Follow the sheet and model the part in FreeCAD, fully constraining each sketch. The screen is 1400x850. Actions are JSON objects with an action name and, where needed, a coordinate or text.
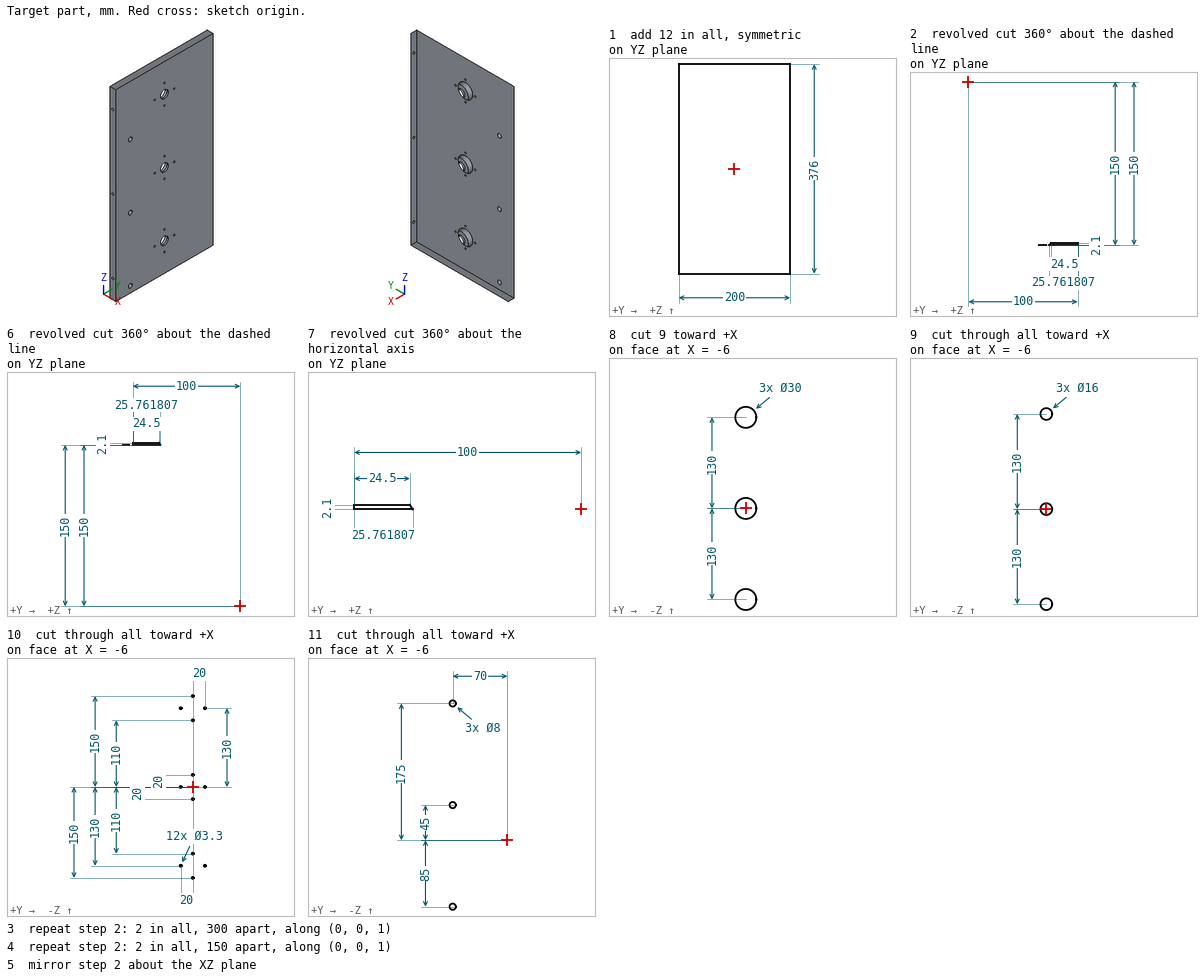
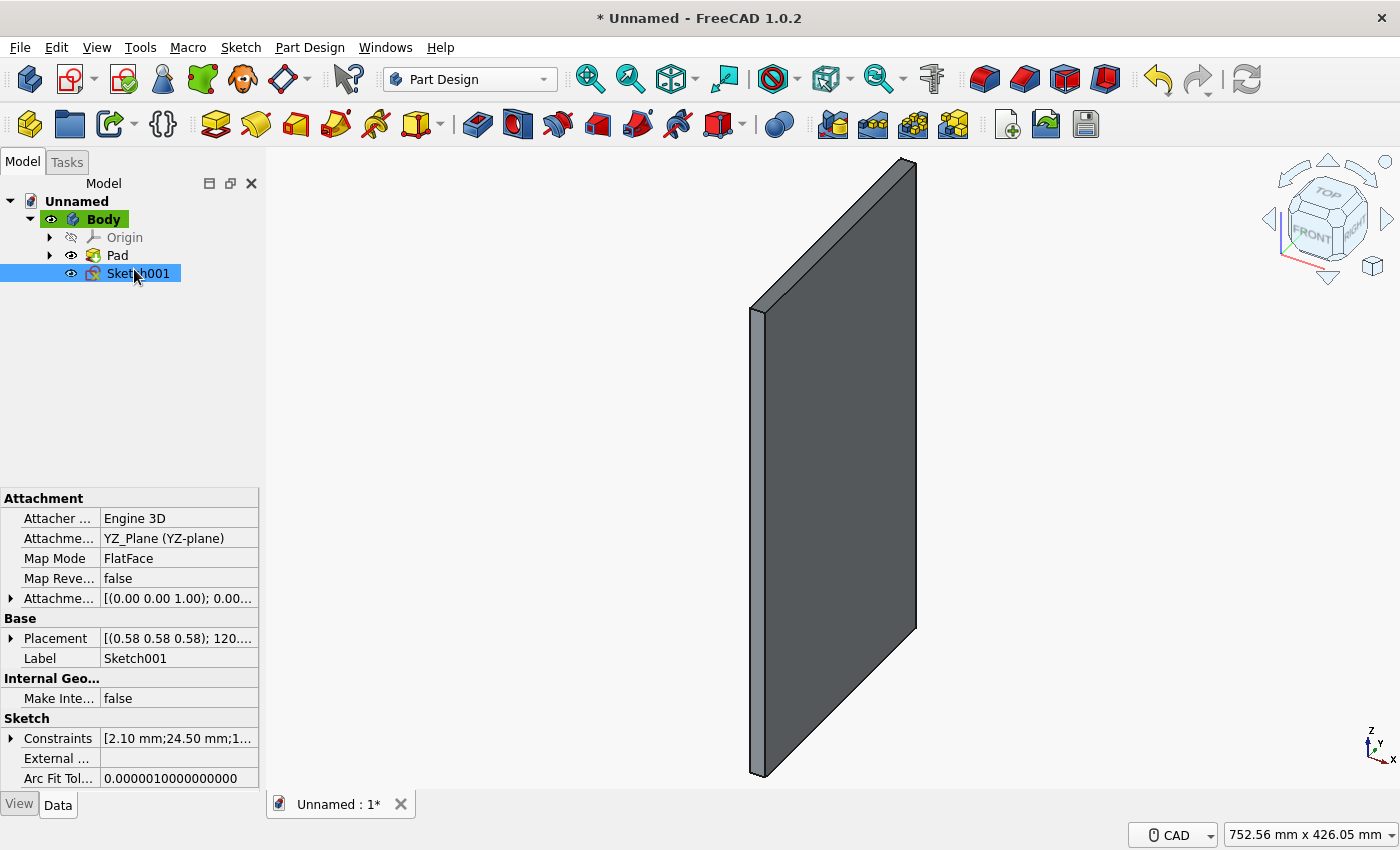
{"action": "left_click", "coordinate": [558, 124]}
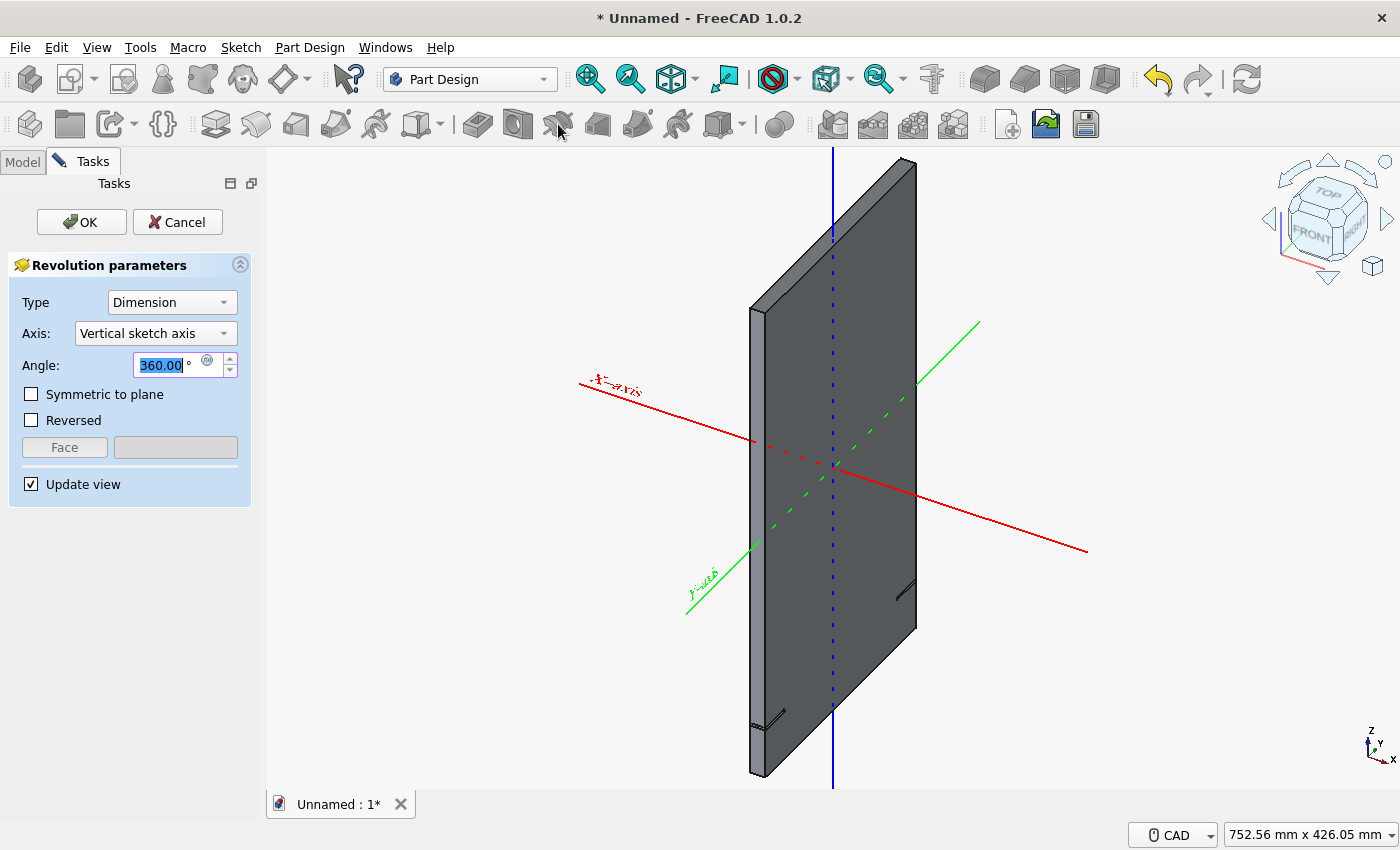
{"action": "left_click", "coordinate": [156, 334]}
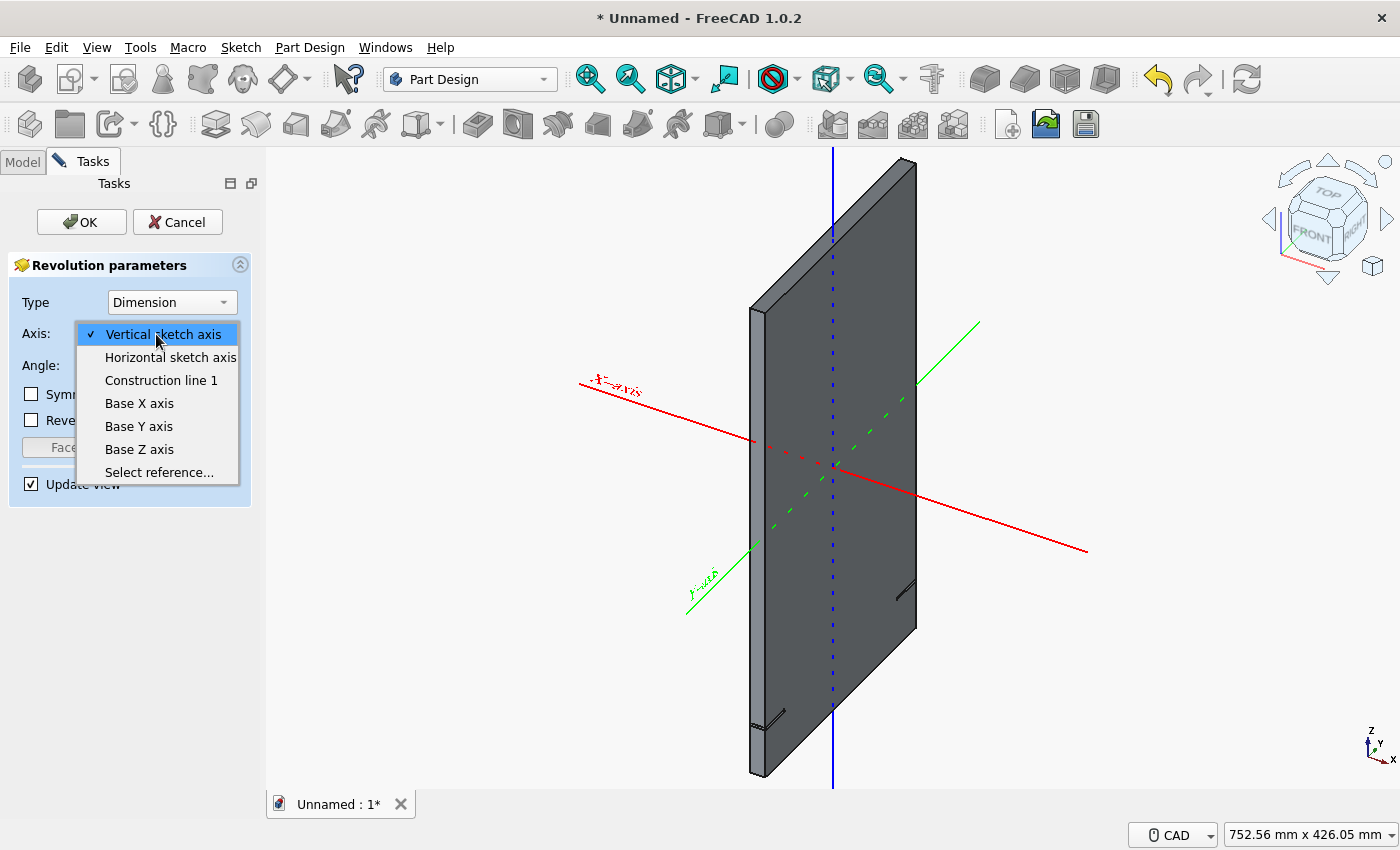
{"action": "left_click", "coordinate": [156, 380]}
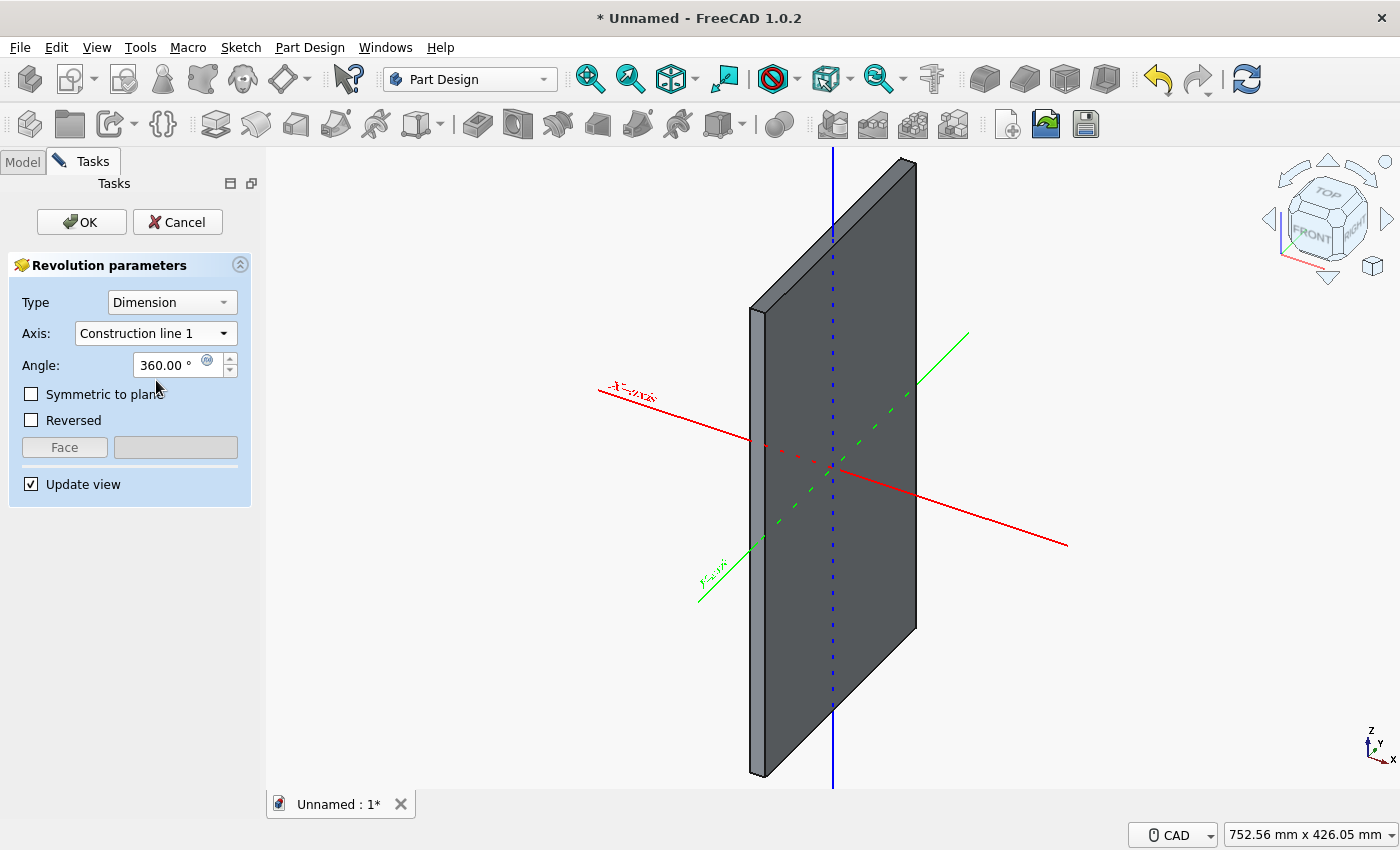
{"action": "left_click", "coordinate": [82, 222]}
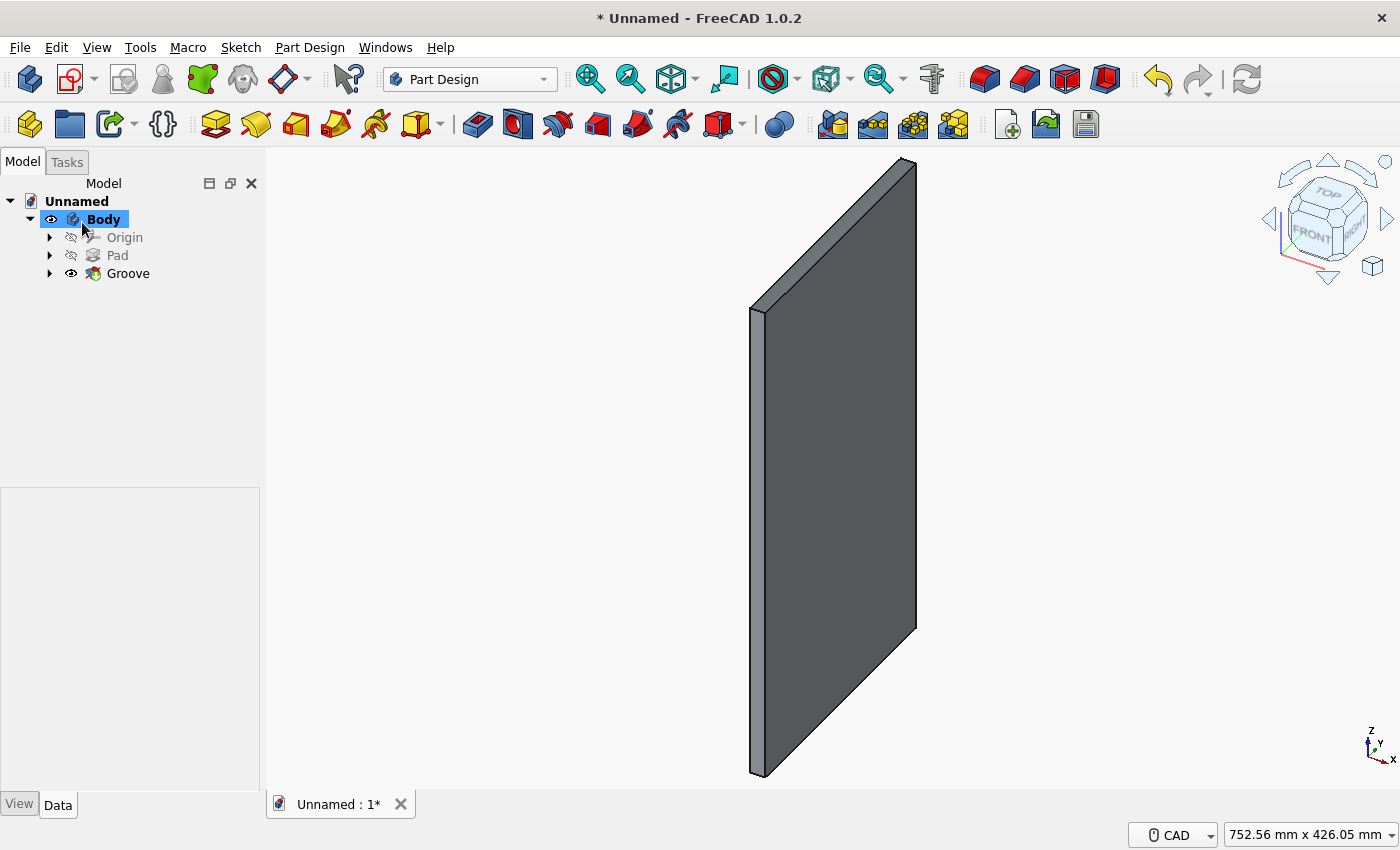
{"action": "left_click", "coordinate": [116, 273]}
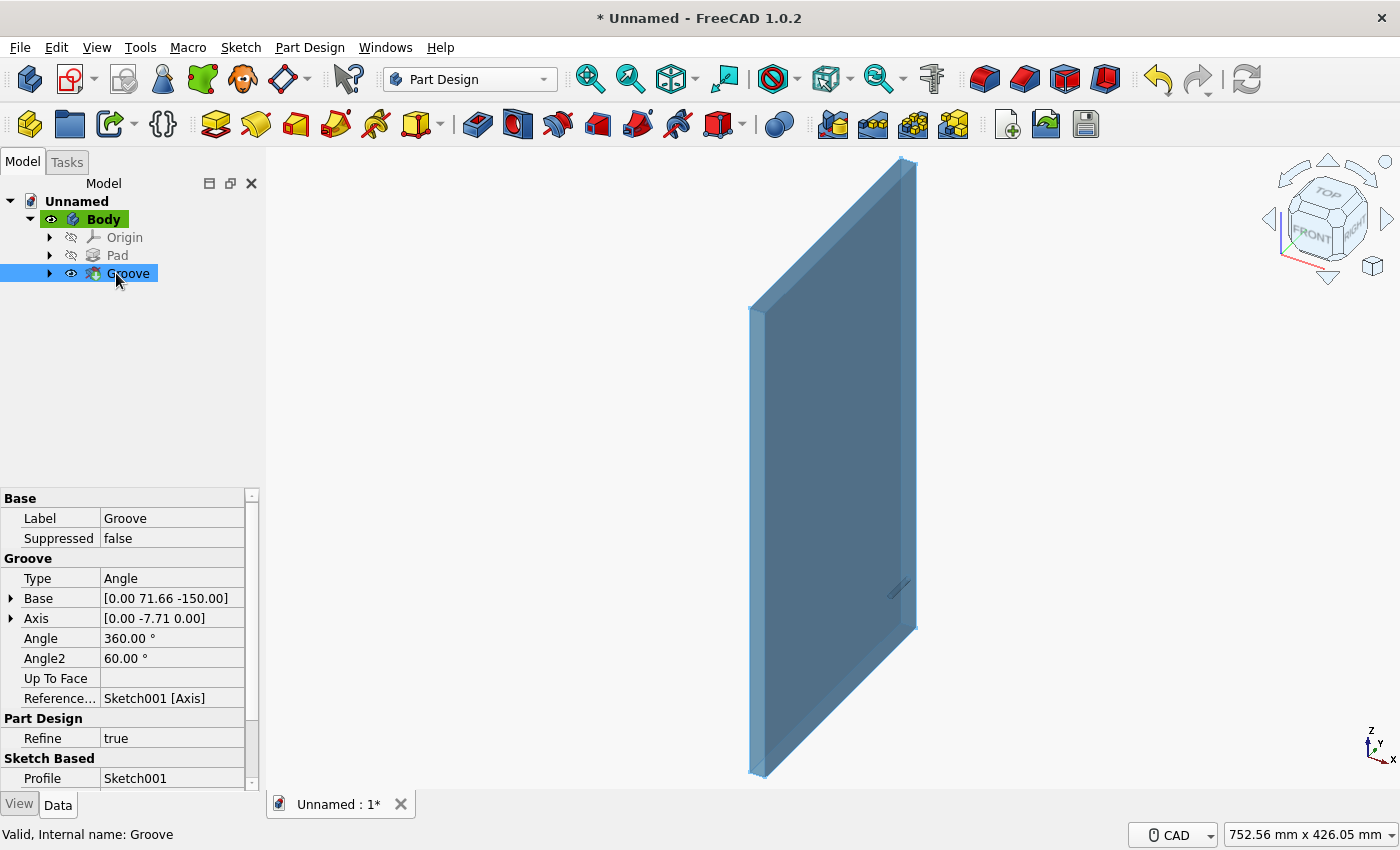
{"action": "left_click", "coordinate": [874, 124]}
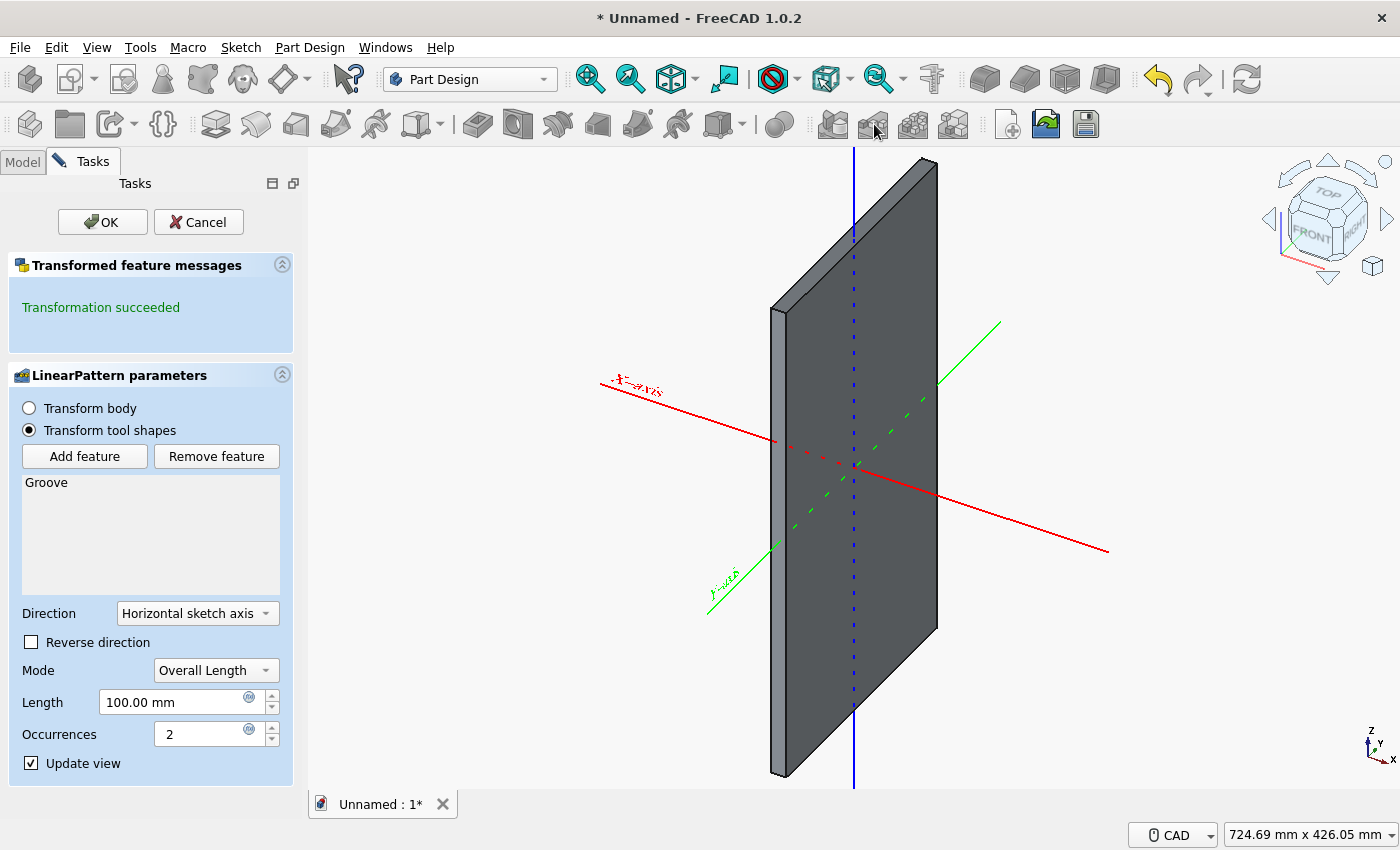
{"action": "left_click", "coordinate": [198, 614]}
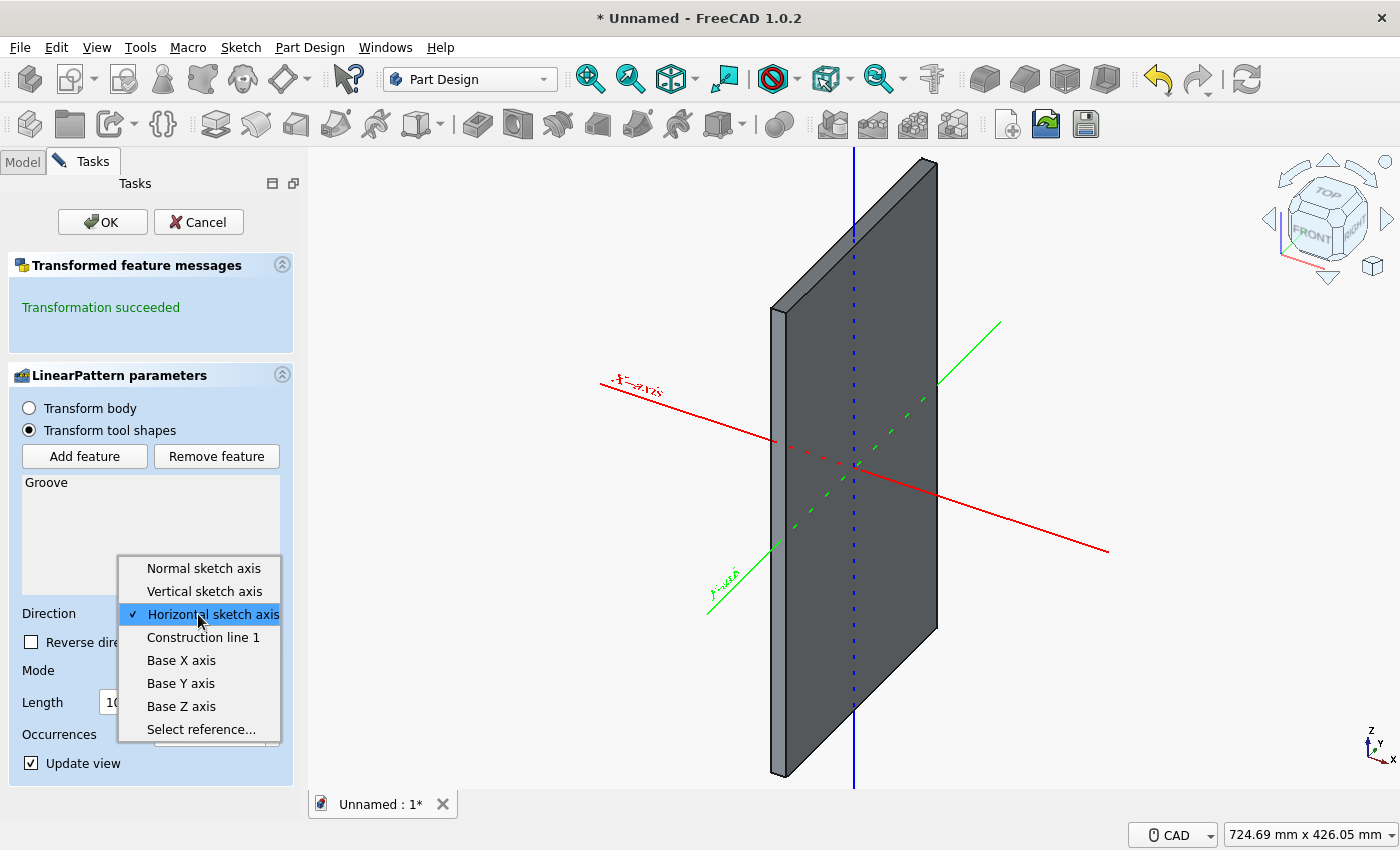
{"action": "left_click", "coordinate": [198, 706]}